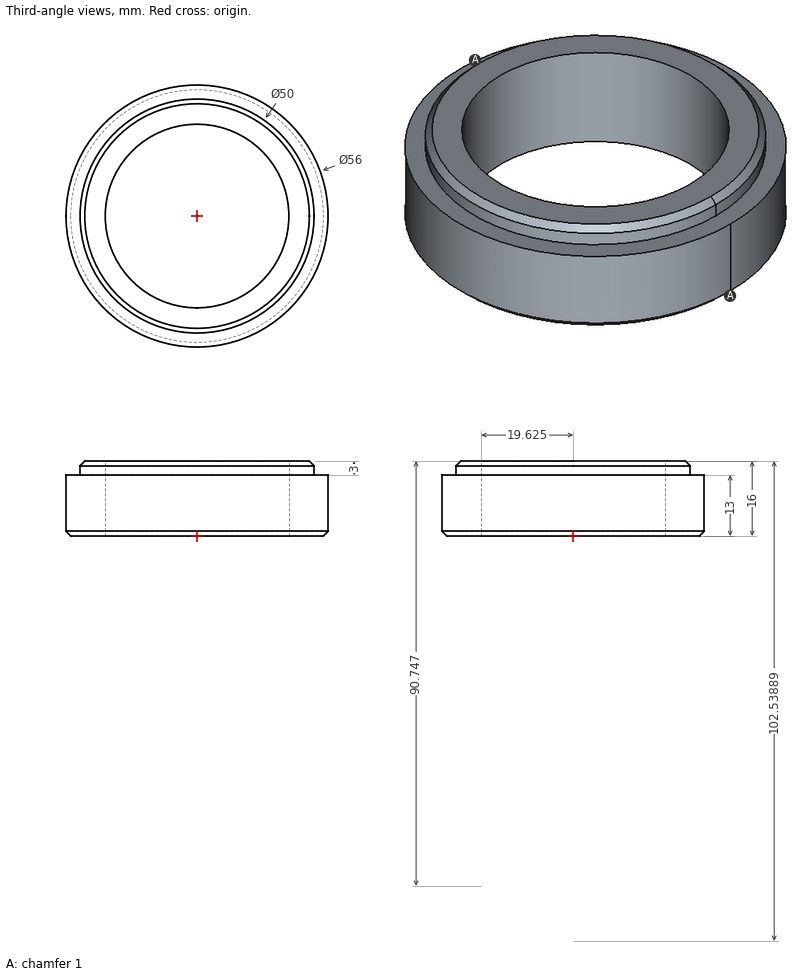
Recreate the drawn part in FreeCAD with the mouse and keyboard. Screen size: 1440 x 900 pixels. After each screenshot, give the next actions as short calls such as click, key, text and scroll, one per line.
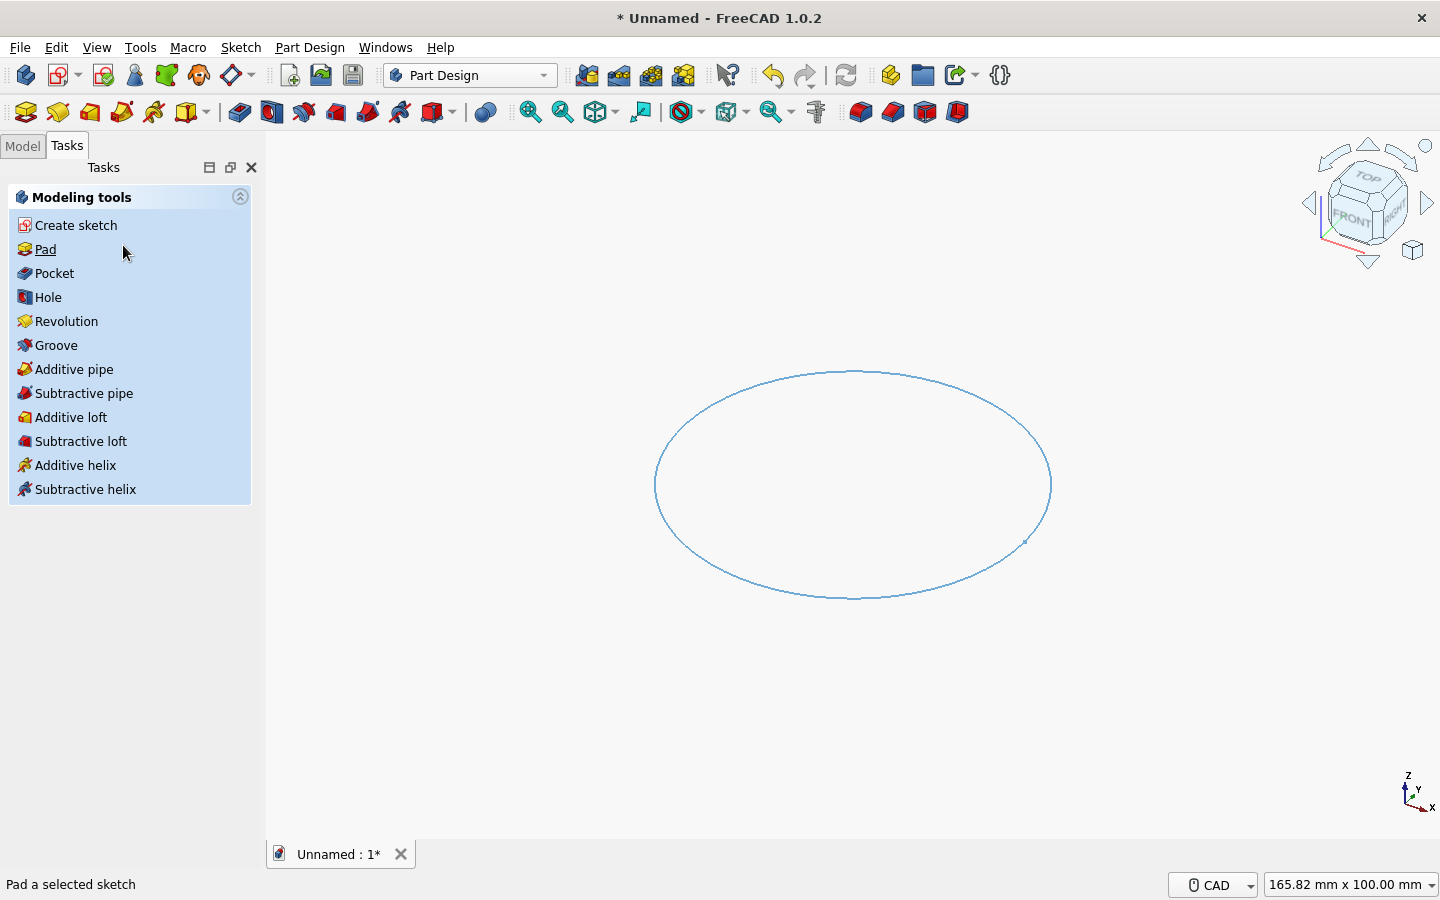
click(26, 112)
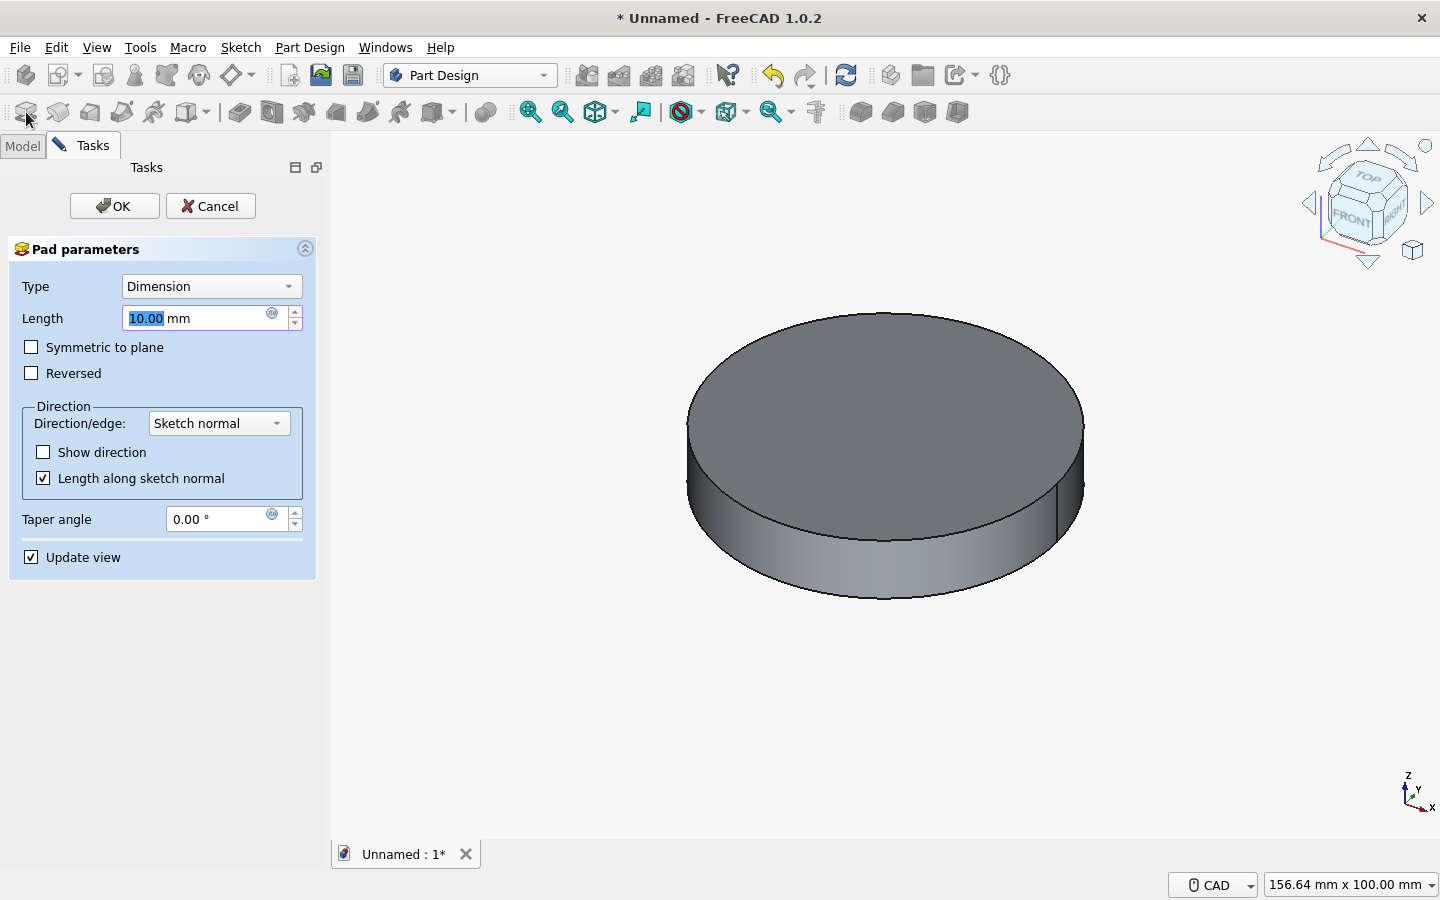
text(13)
key(Tab)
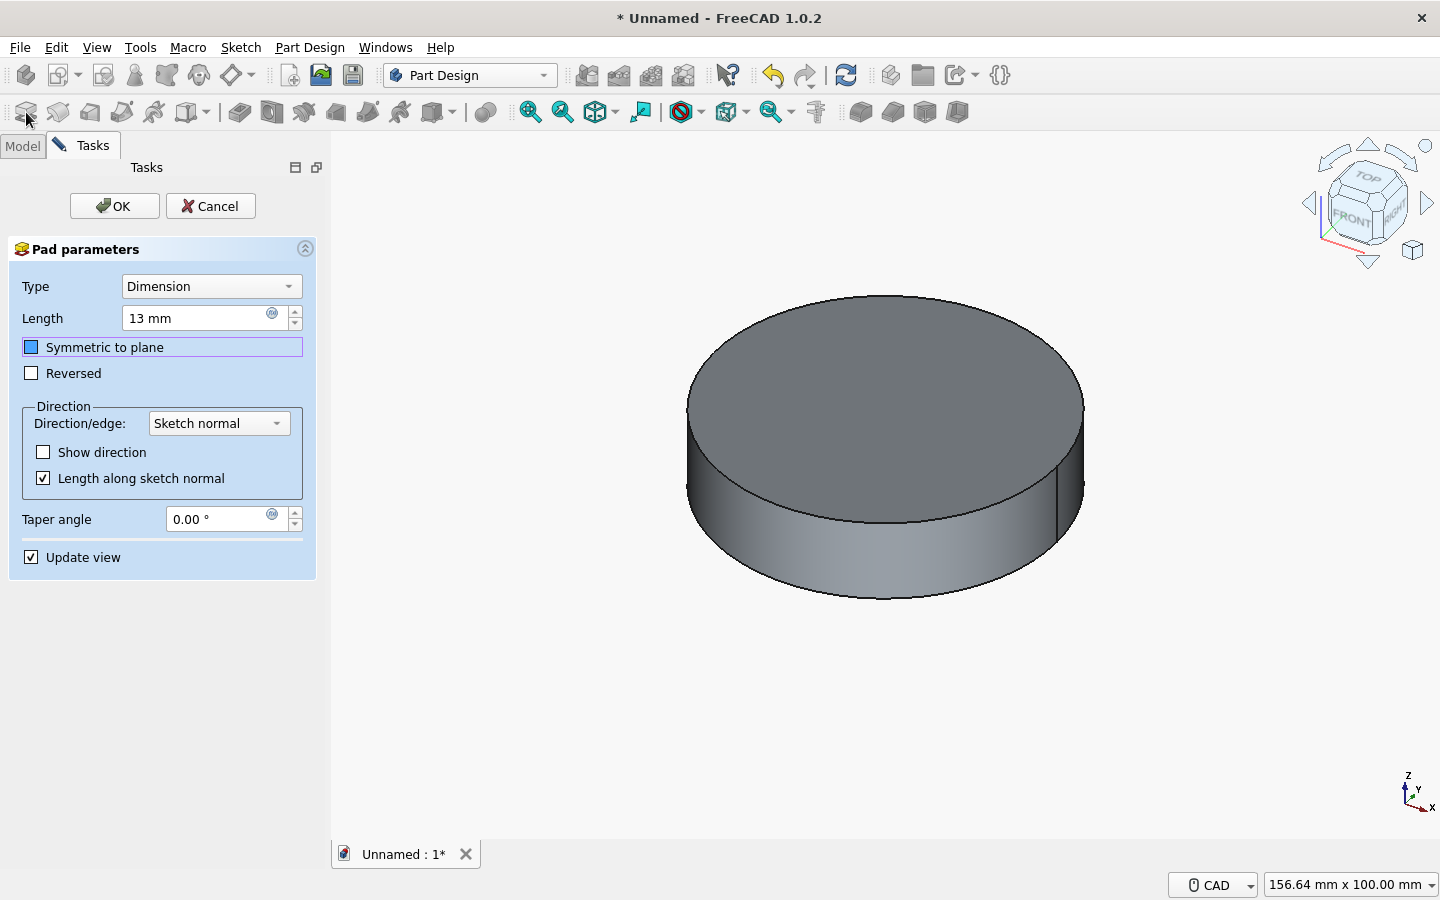
click(115, 206)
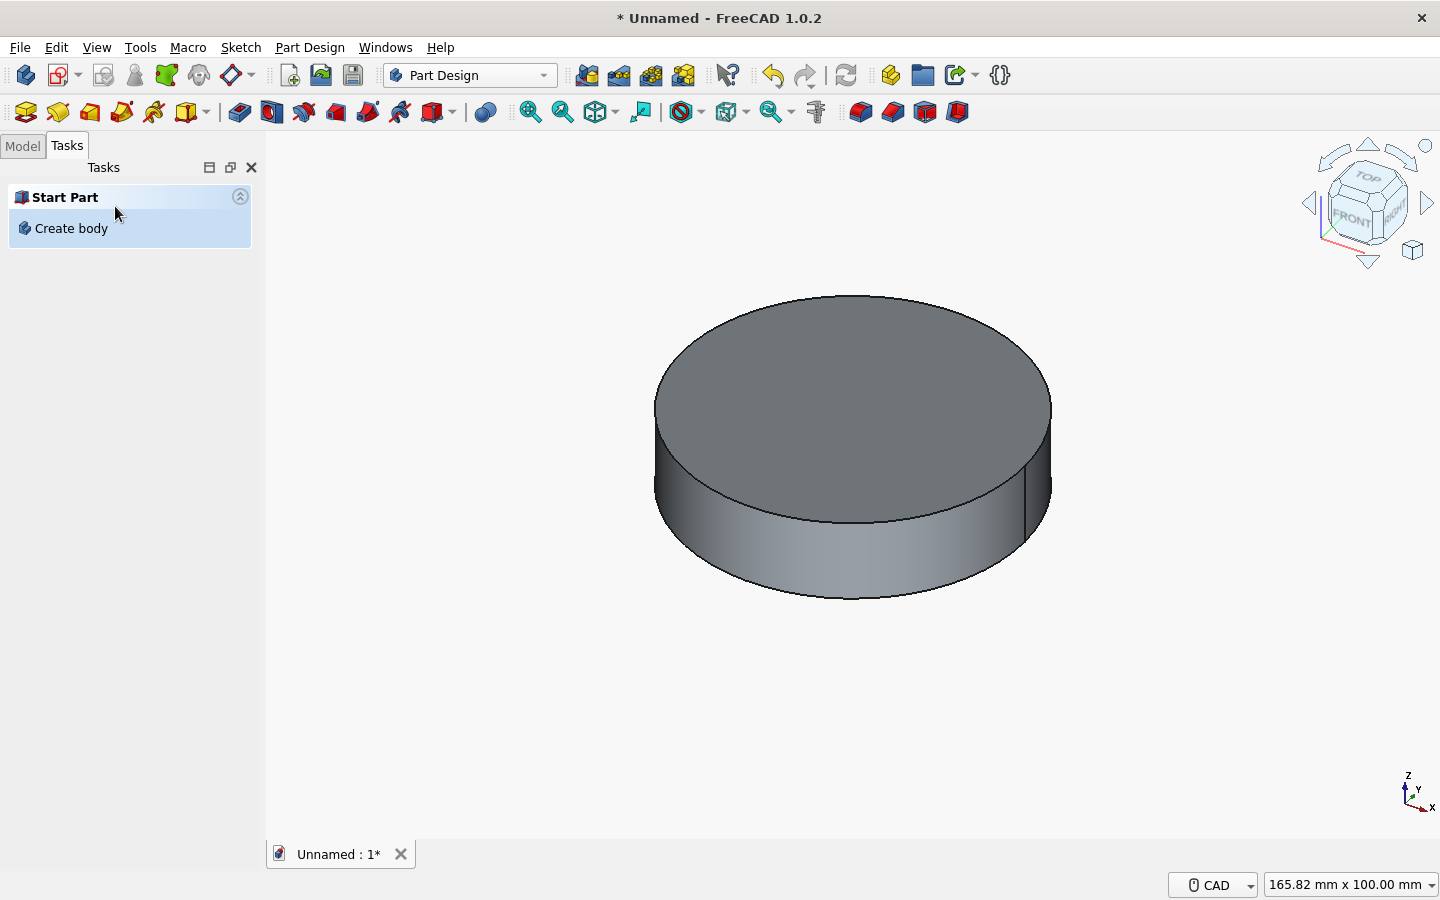
click(853, 409)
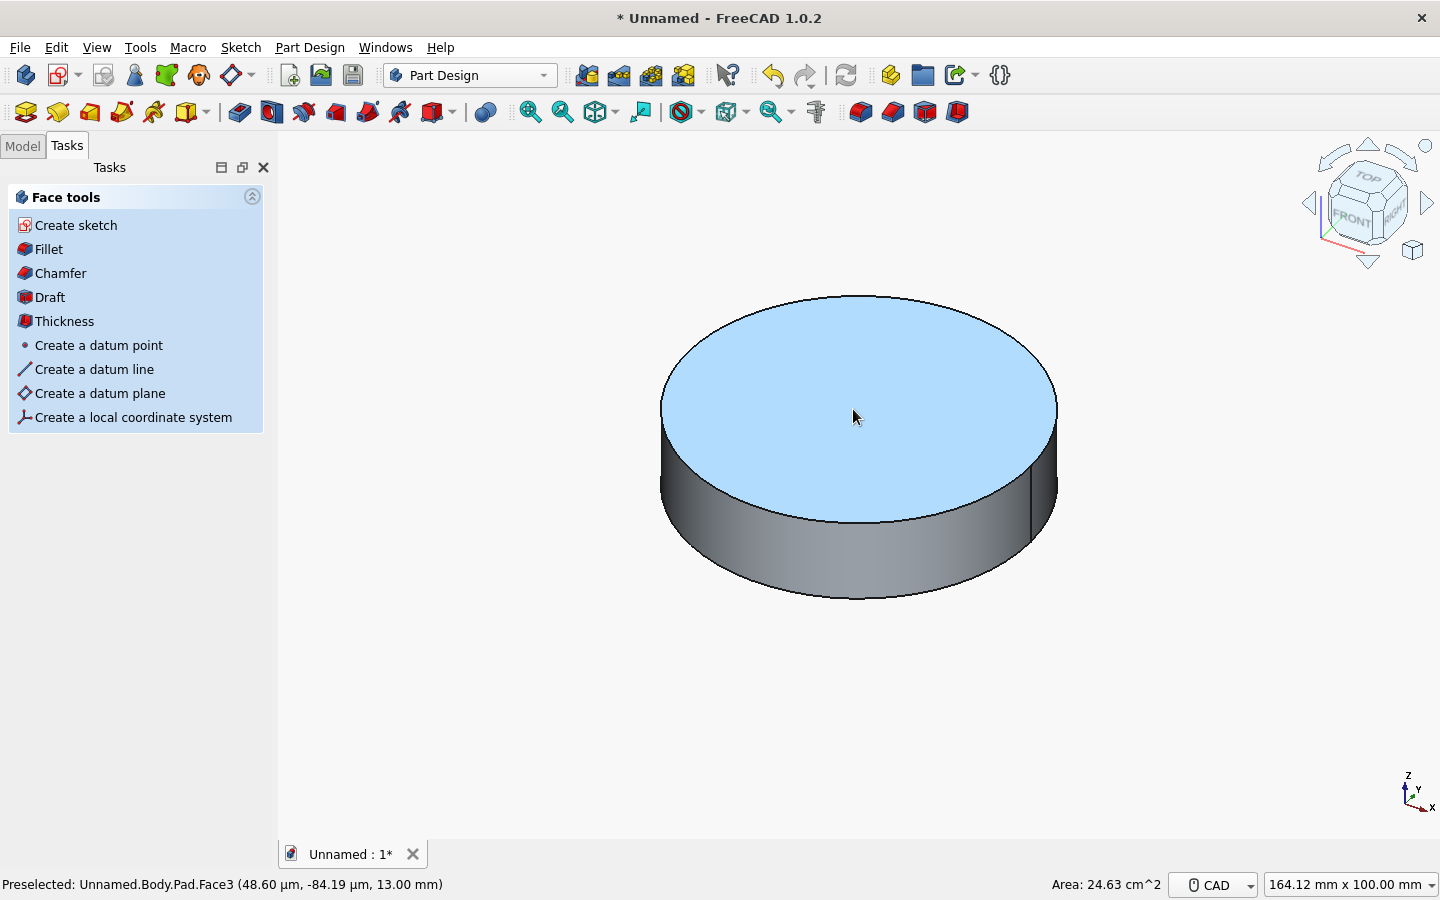
click(58, 76)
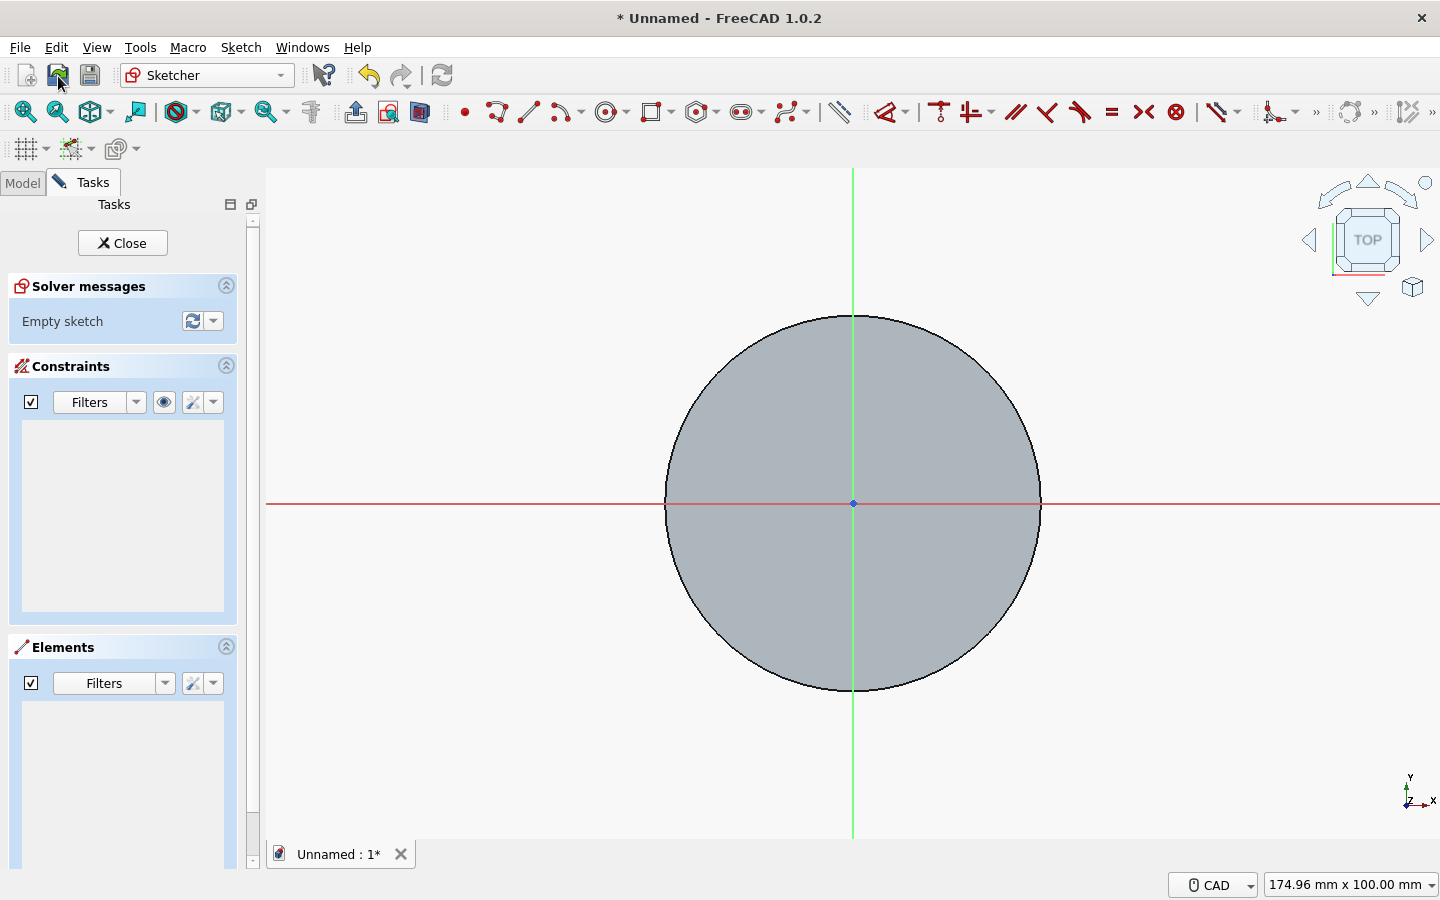
click(606, 112)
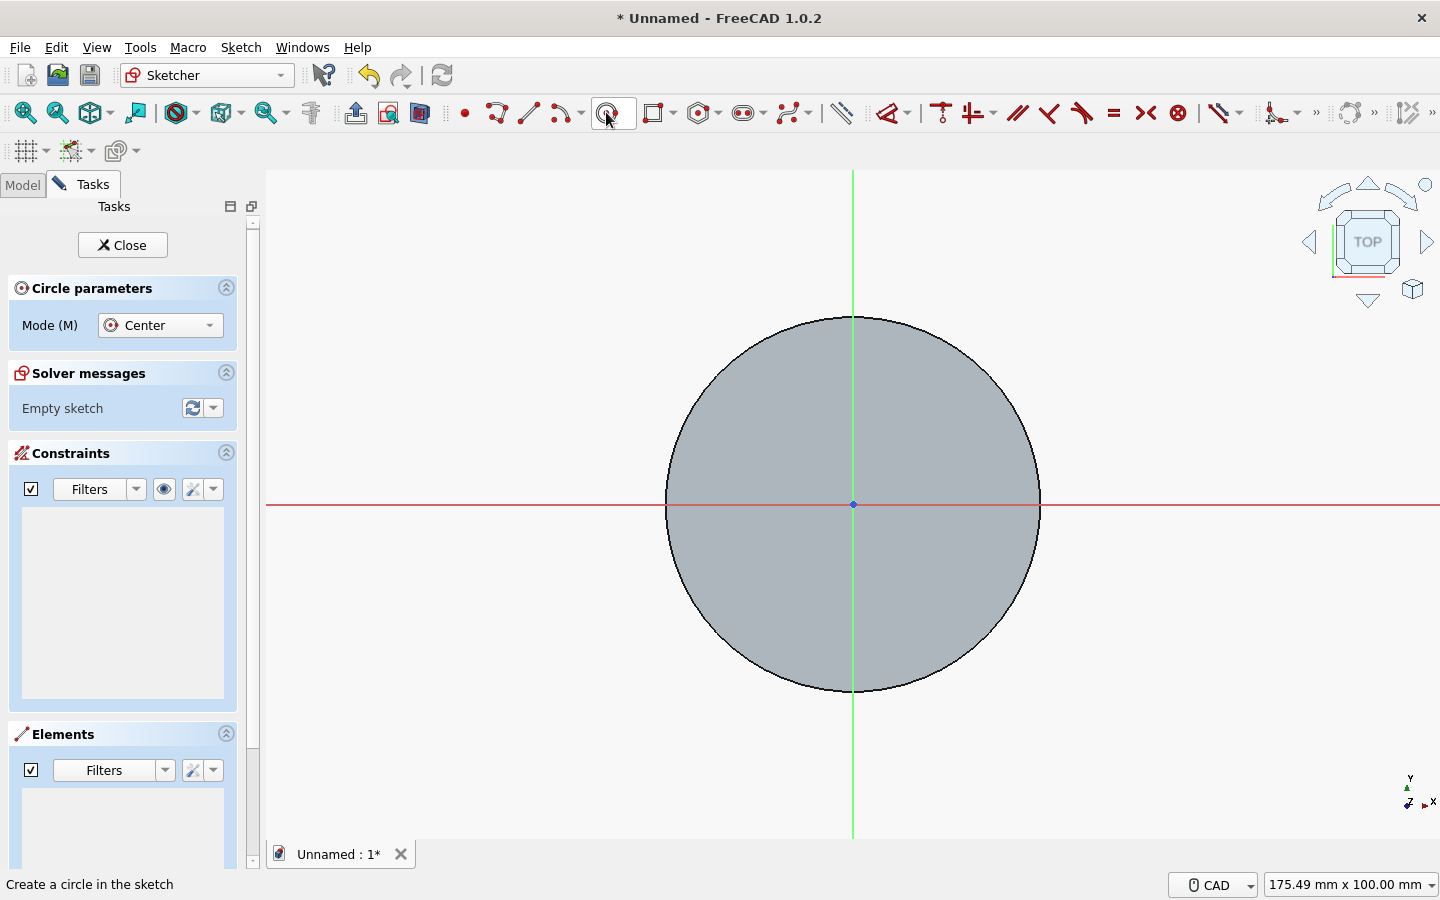
click(853, 504)
move(971, 386)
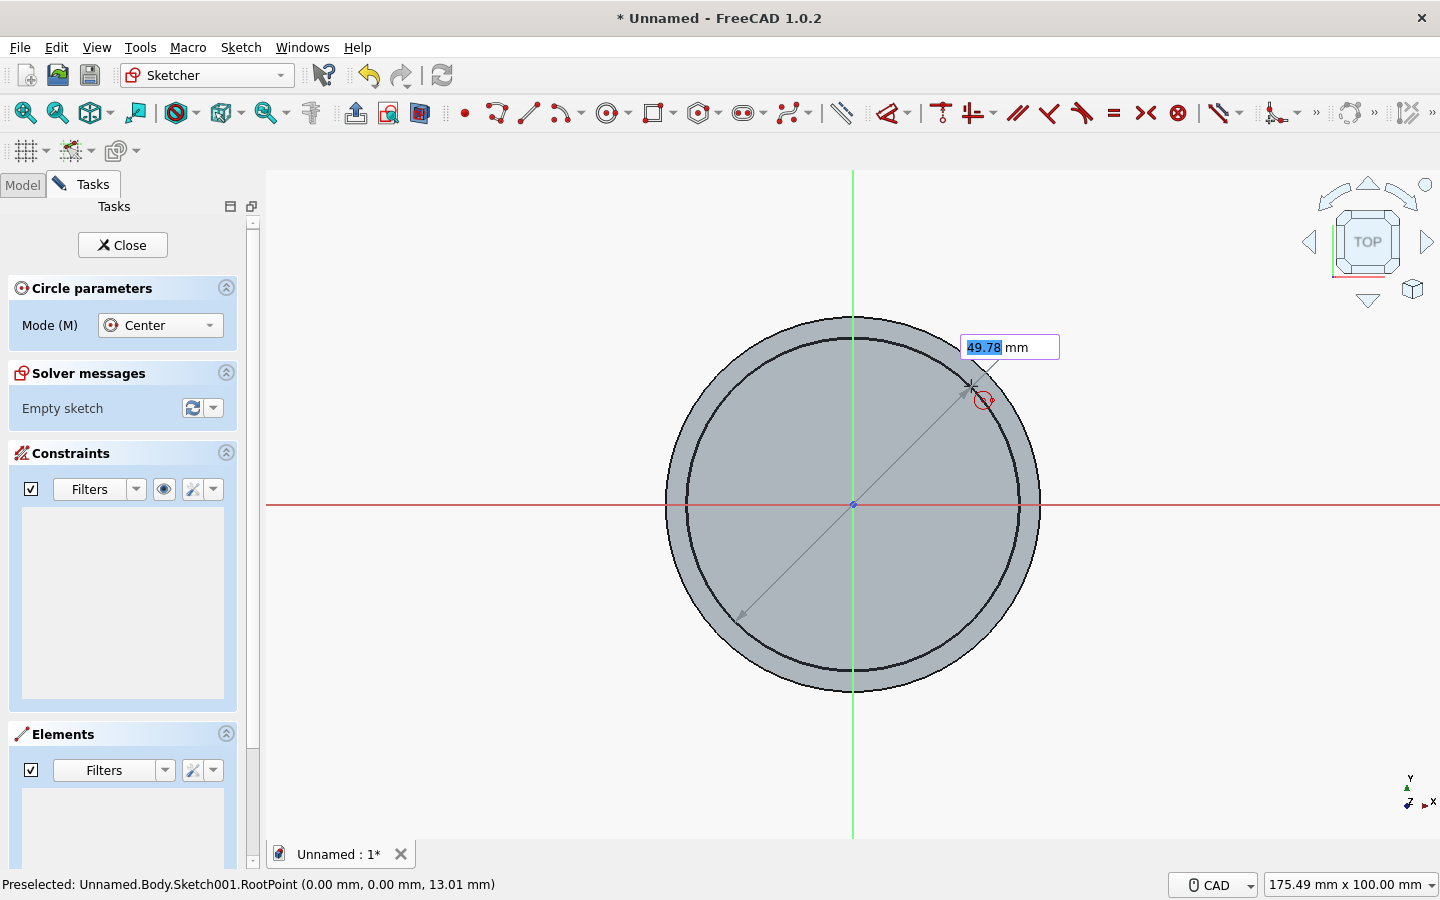
text(50)
key(Return)
key(Escape)